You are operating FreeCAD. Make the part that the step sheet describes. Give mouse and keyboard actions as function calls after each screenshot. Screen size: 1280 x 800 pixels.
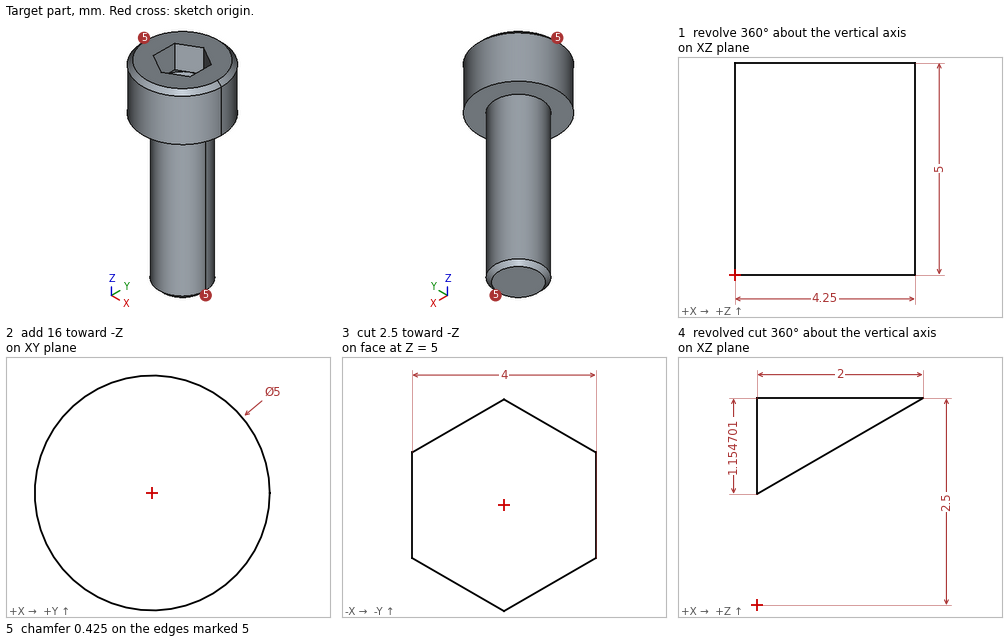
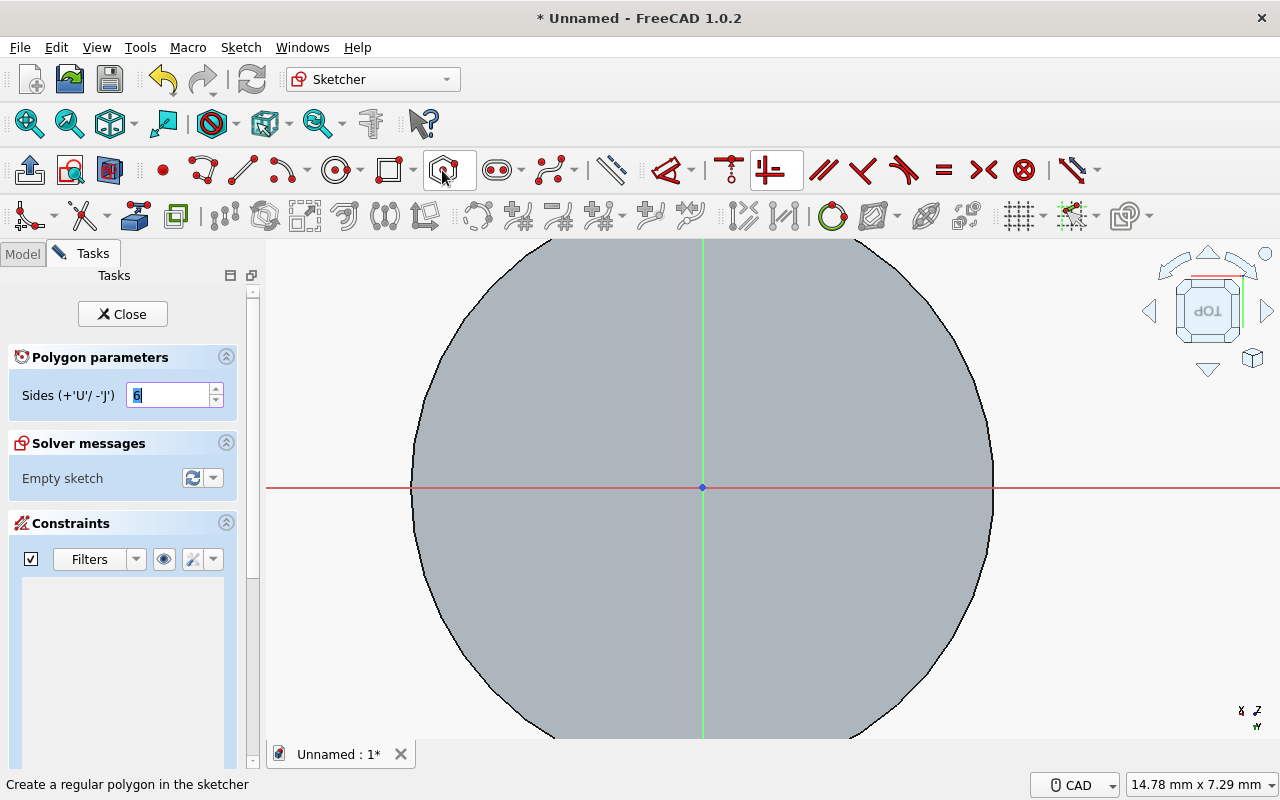
click(703, 488)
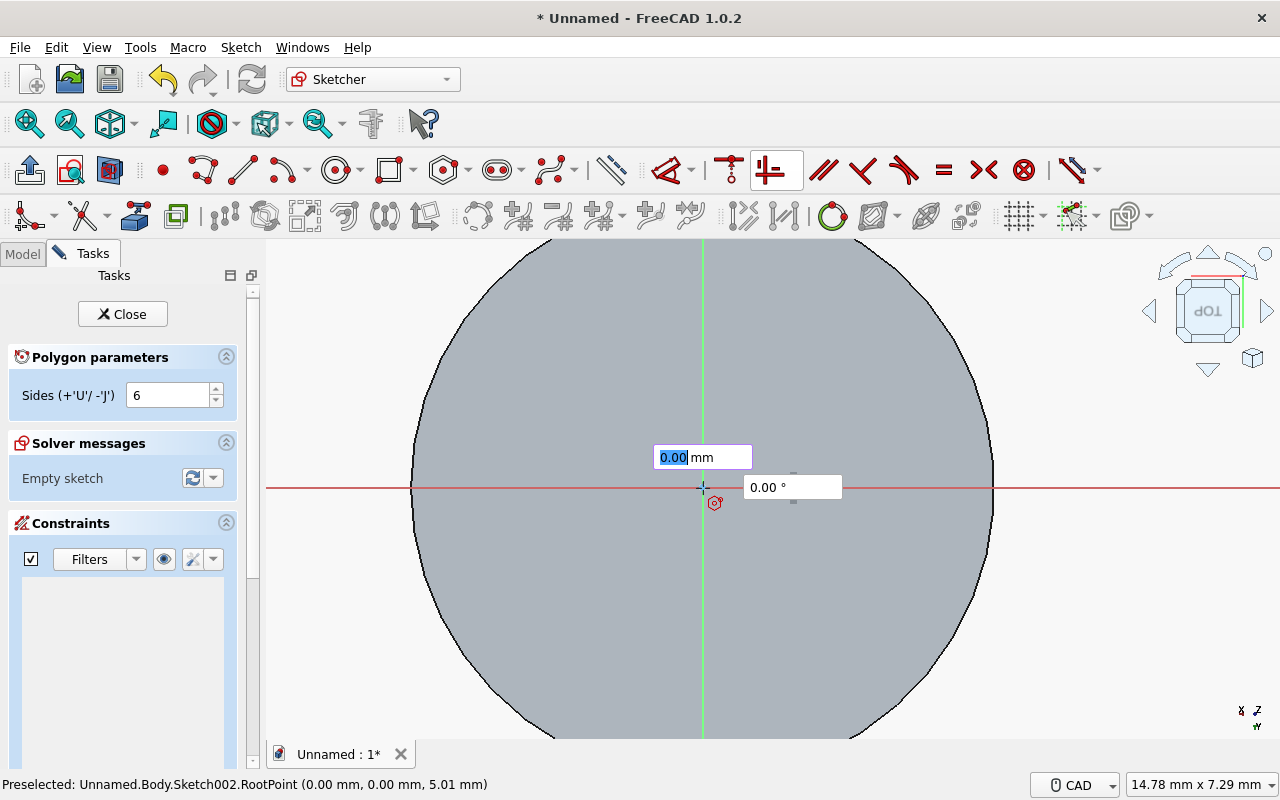
click(703, 646)
right_click(703, 646)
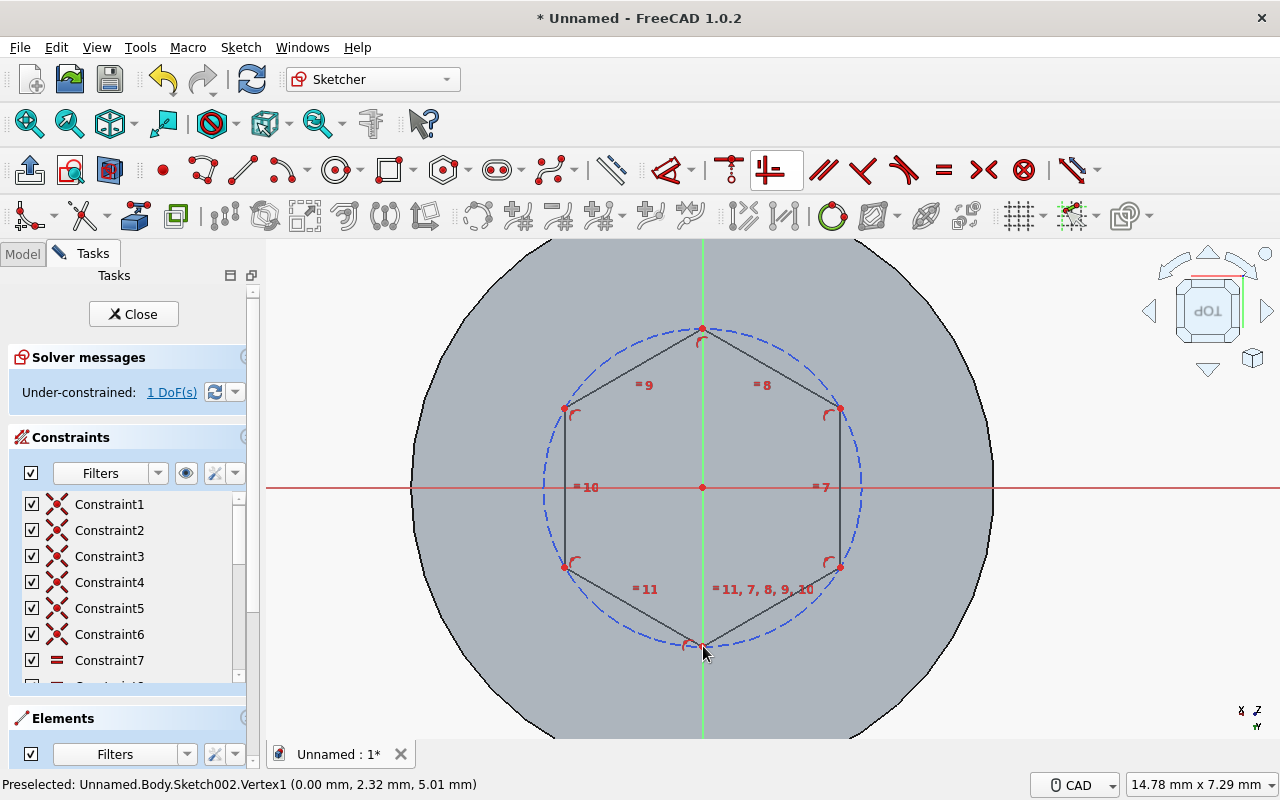
click(565, 408)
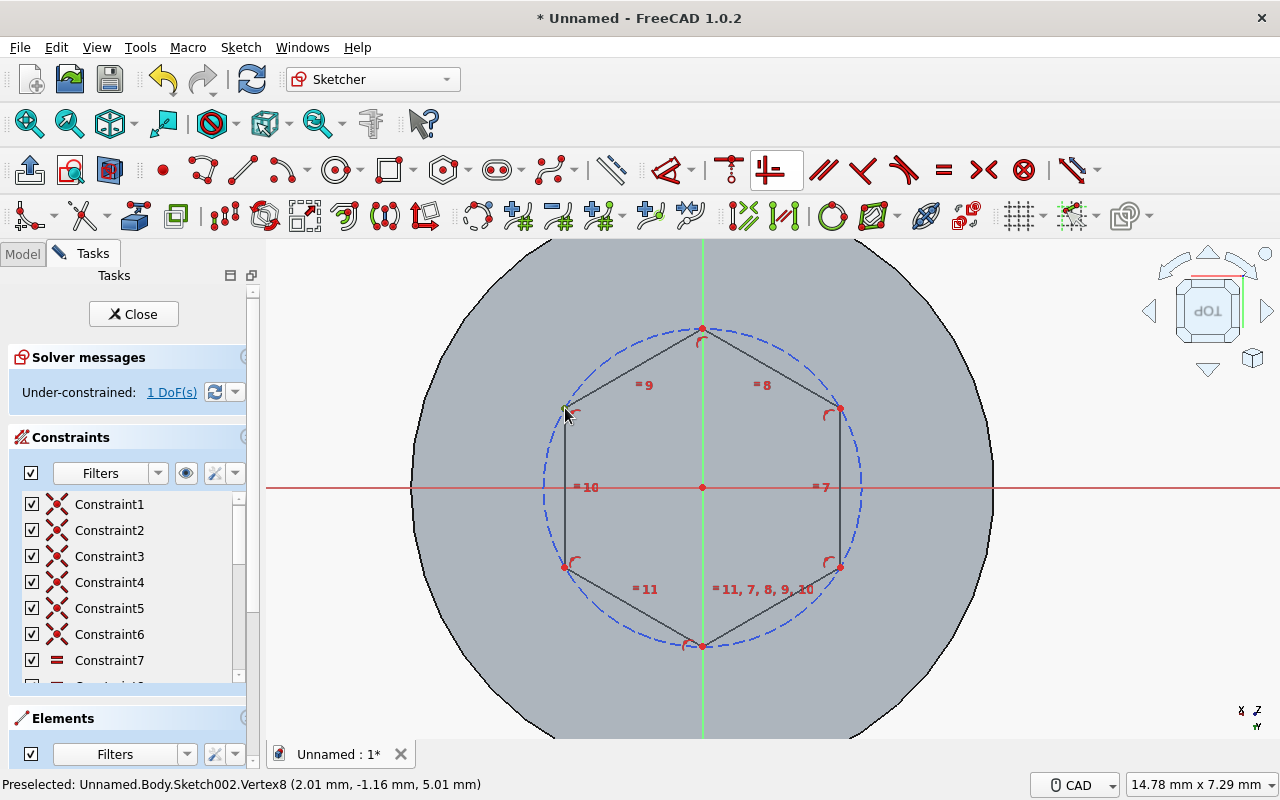
click(840, 567)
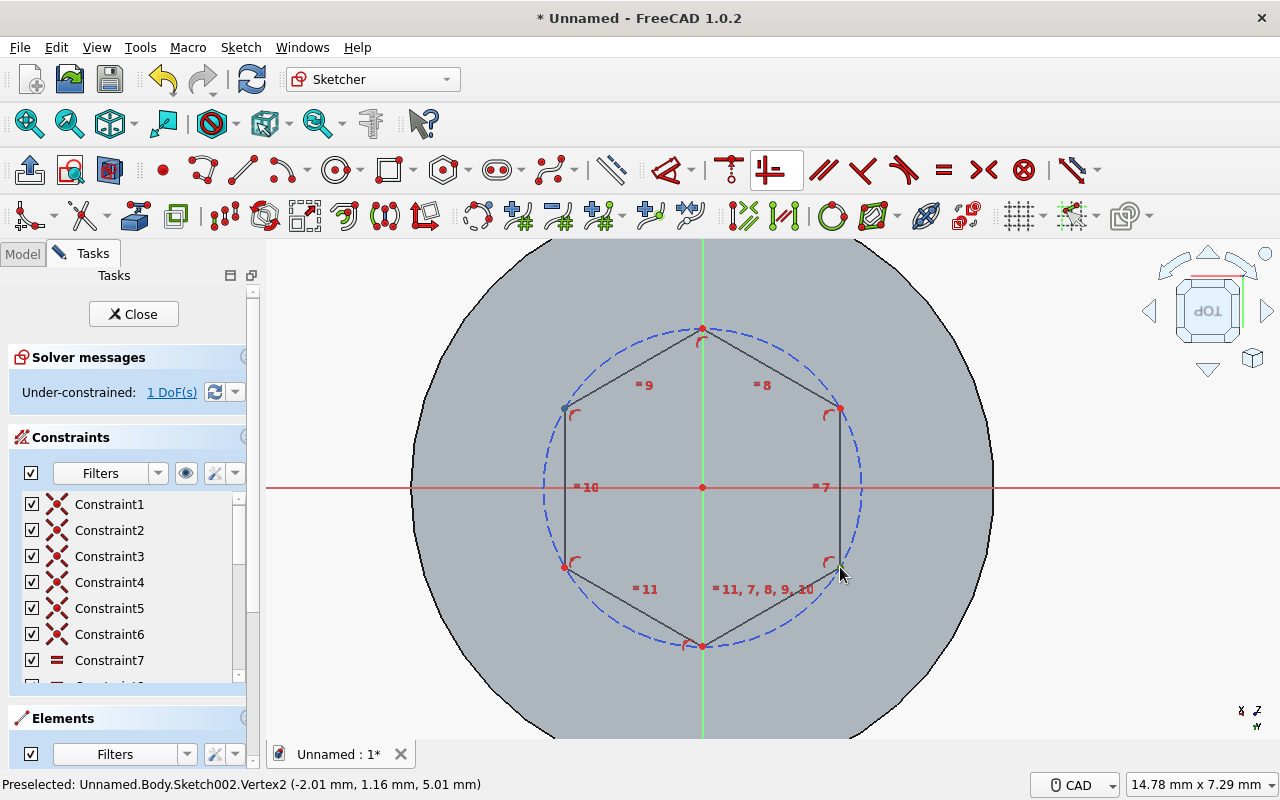
click(694, 170)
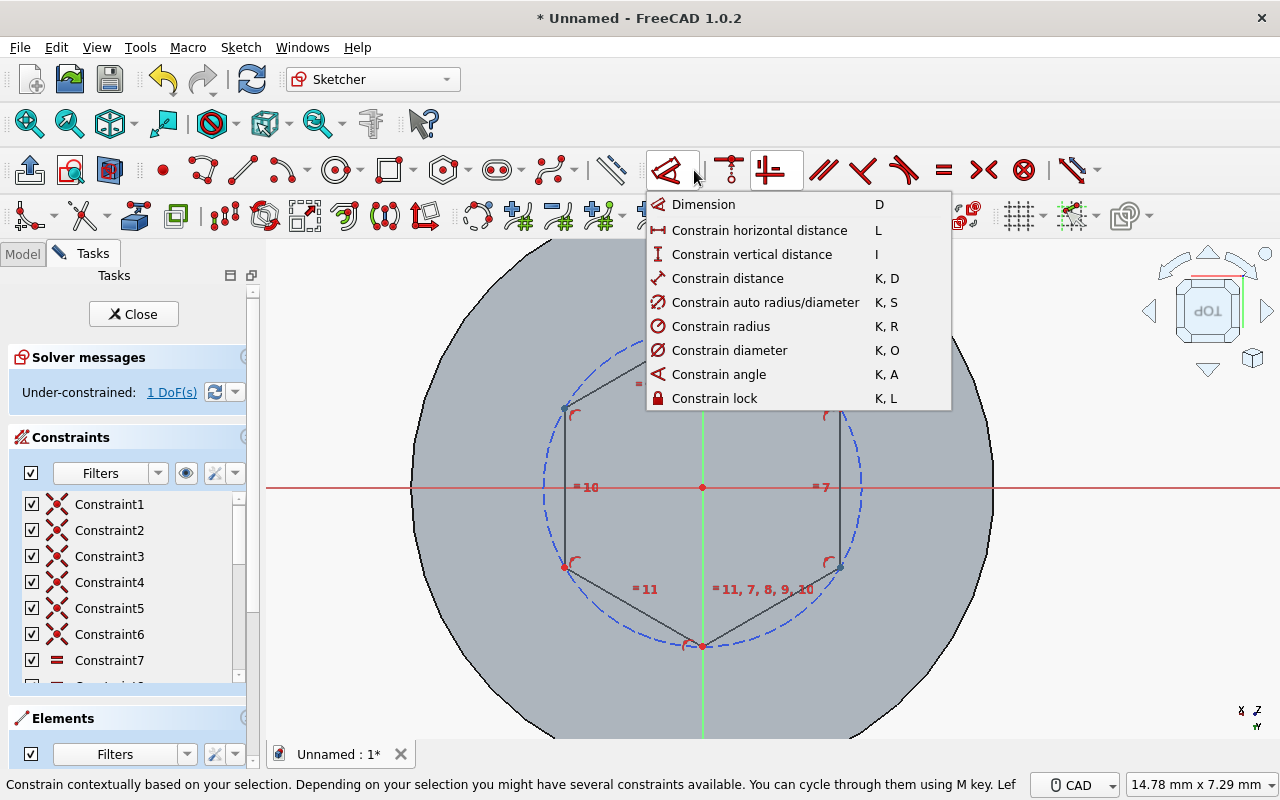
click(799, 230)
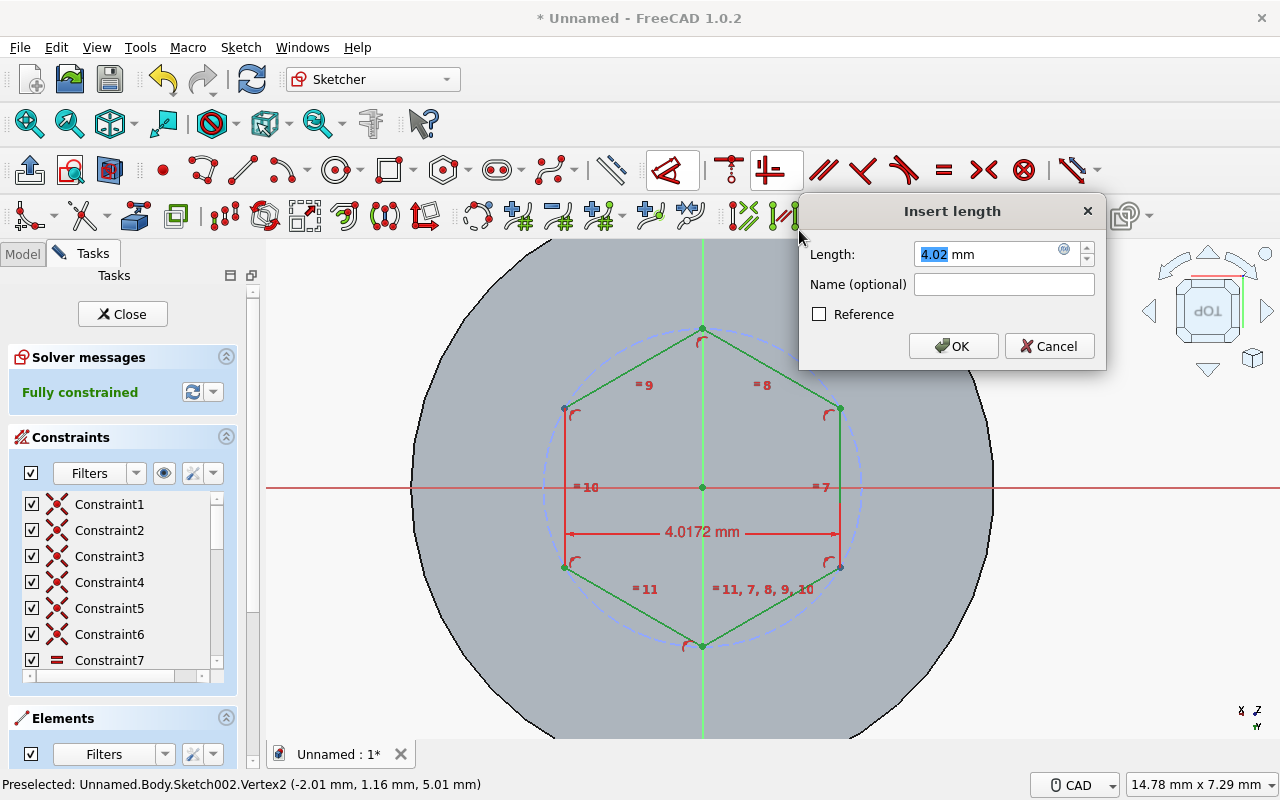
text(4)
key(Return)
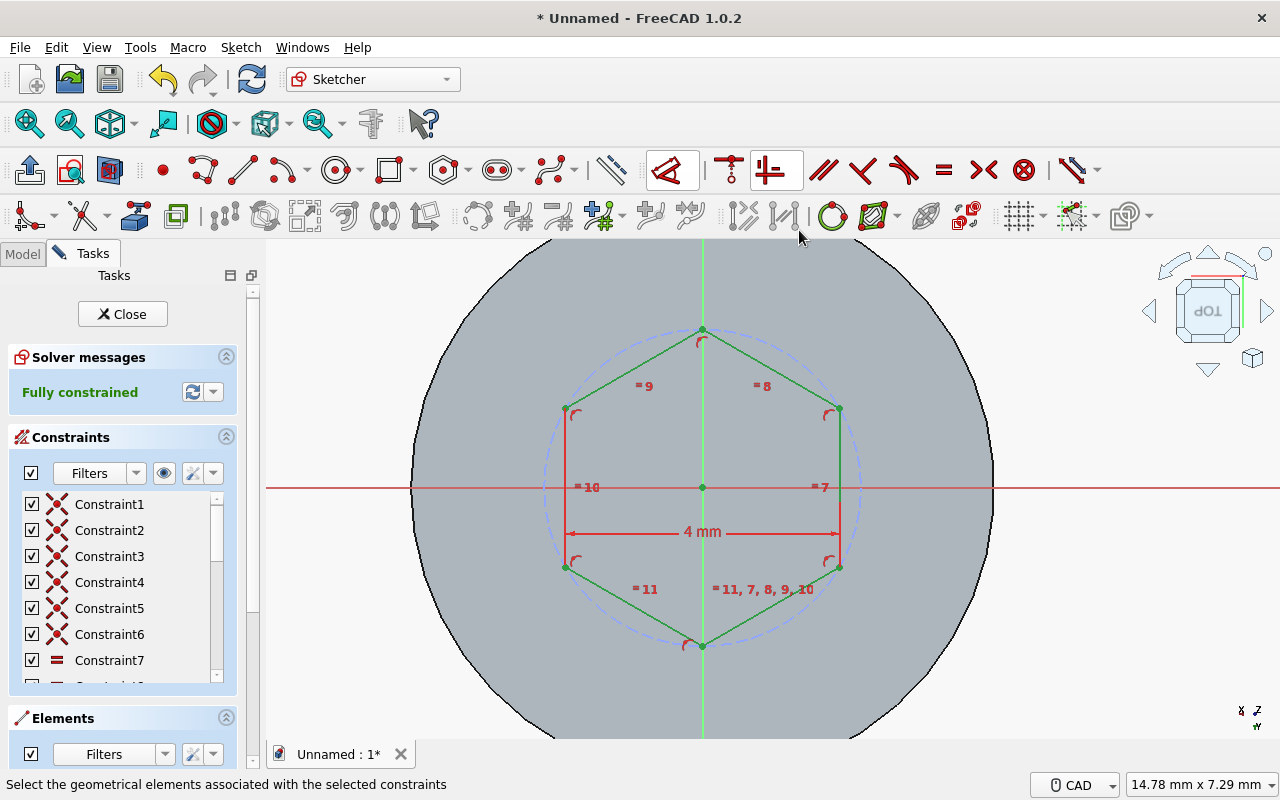
click(123, 314)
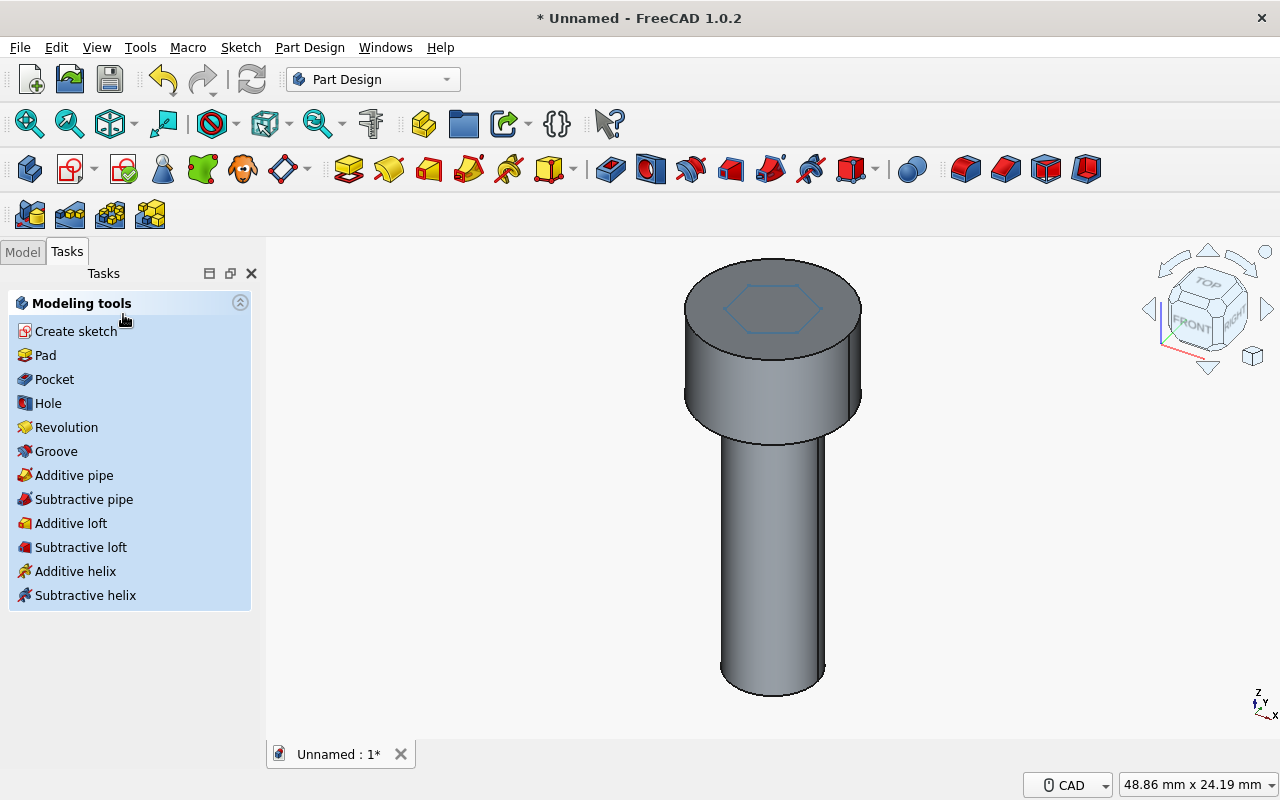
click(612, 170)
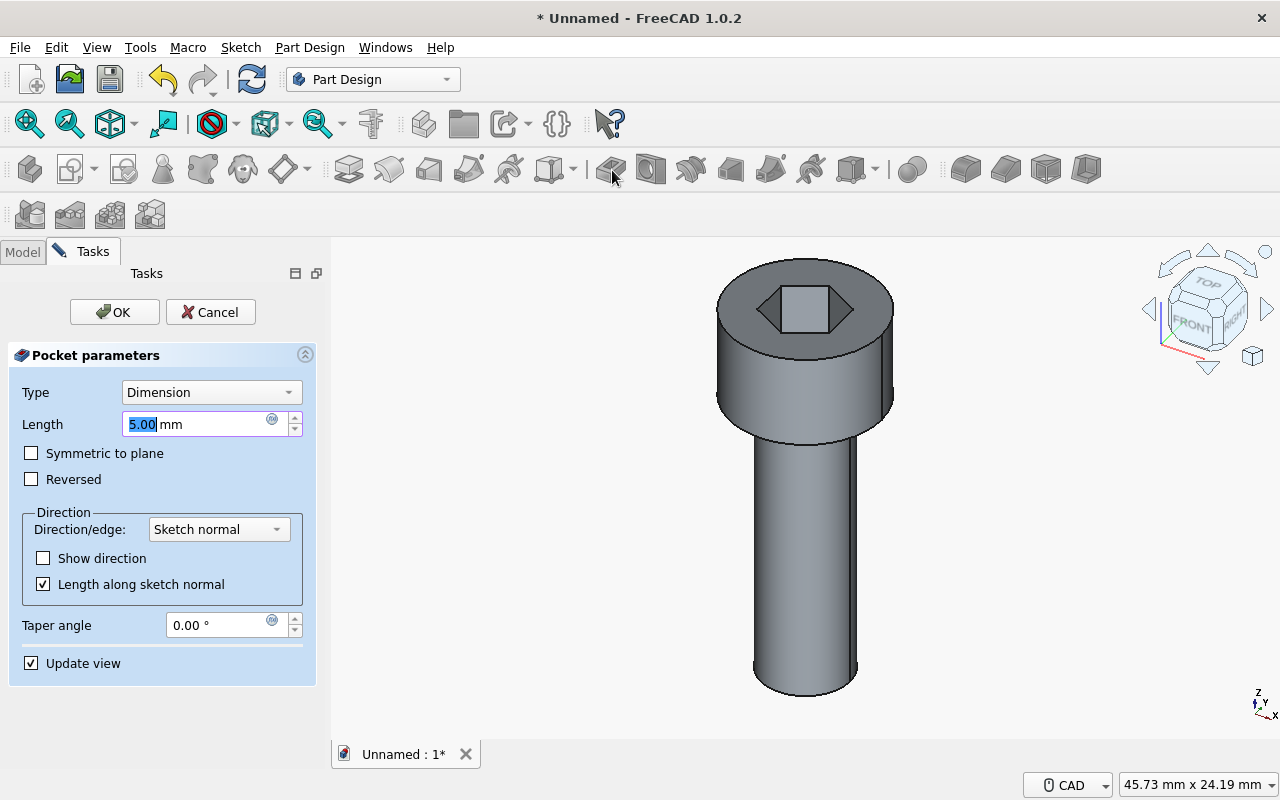
text(2.5)
key(Tab)